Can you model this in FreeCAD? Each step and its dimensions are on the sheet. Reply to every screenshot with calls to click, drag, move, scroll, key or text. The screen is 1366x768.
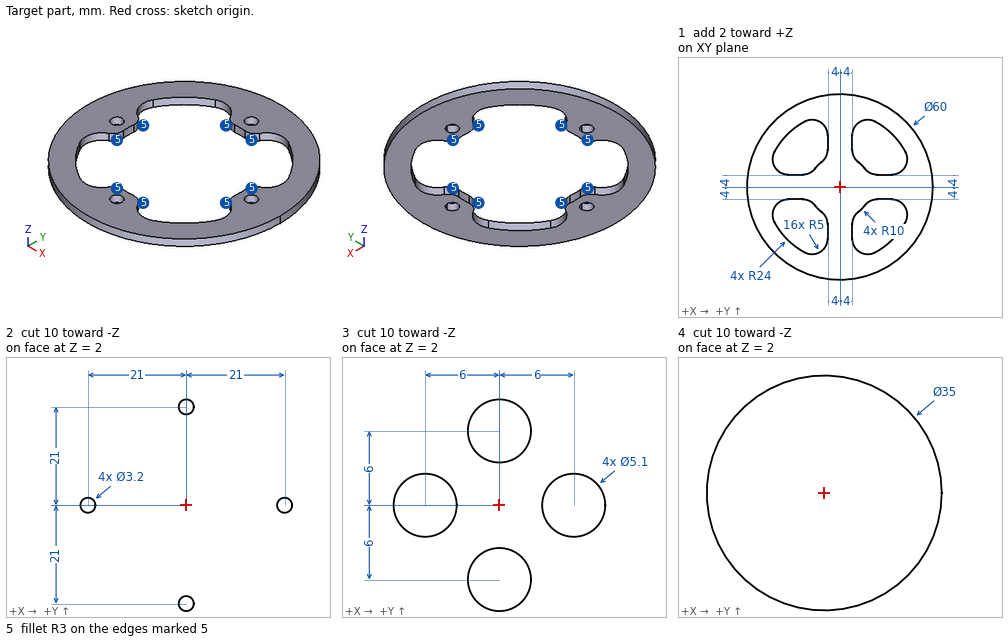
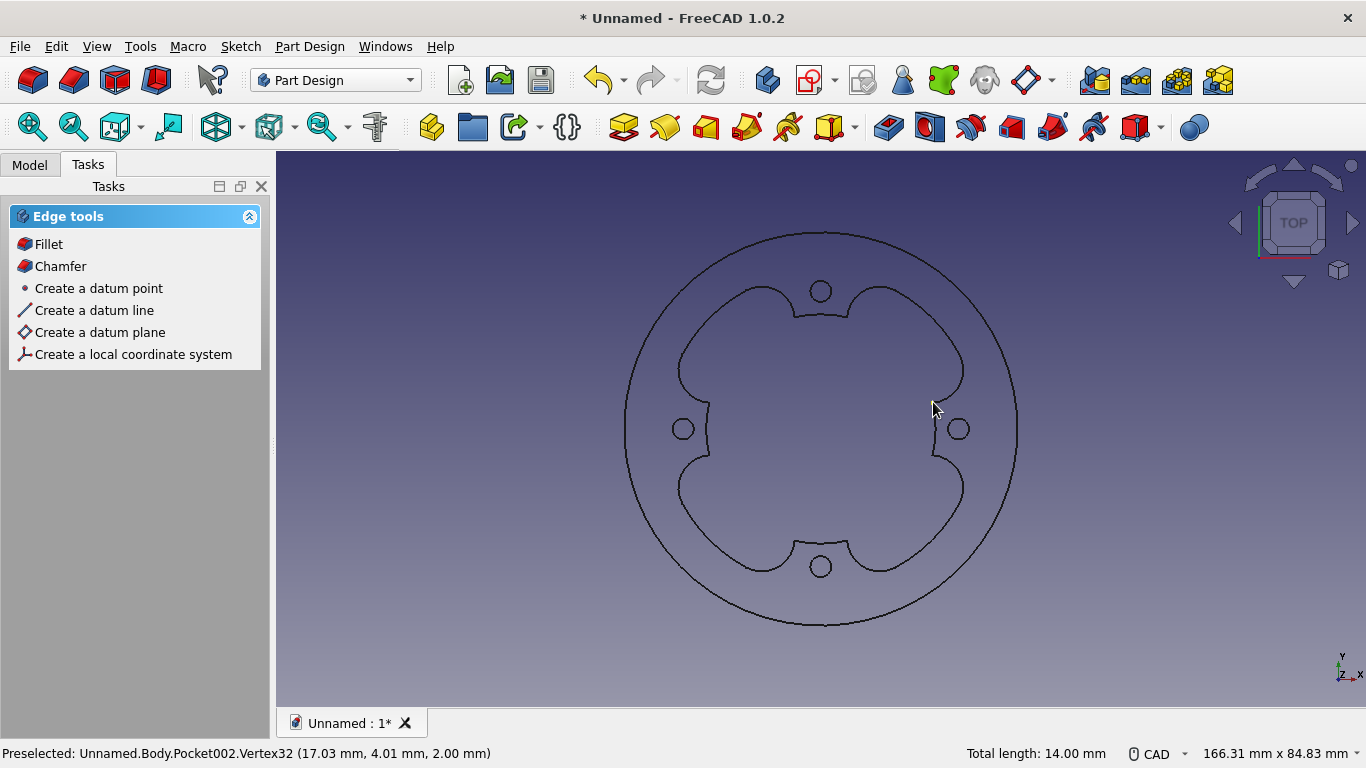
key(1)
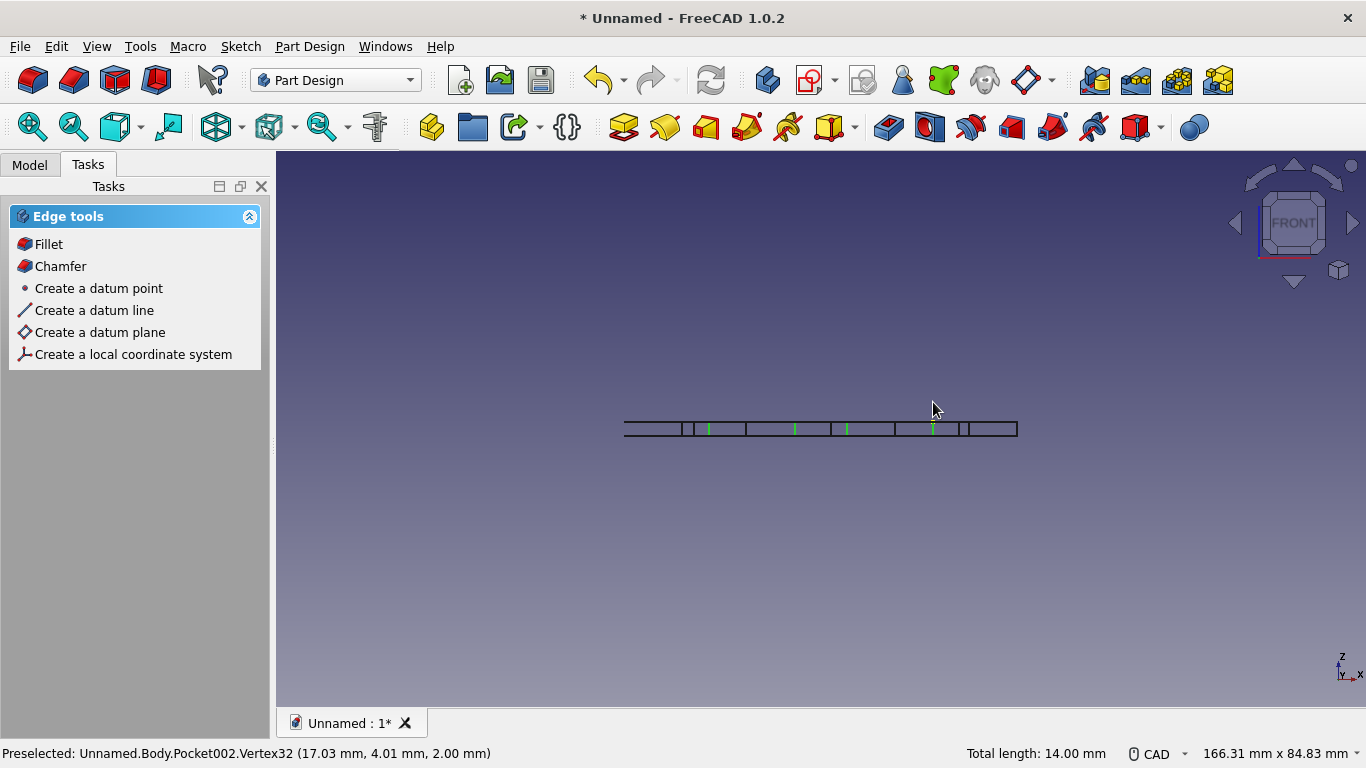
key(v)
key(f)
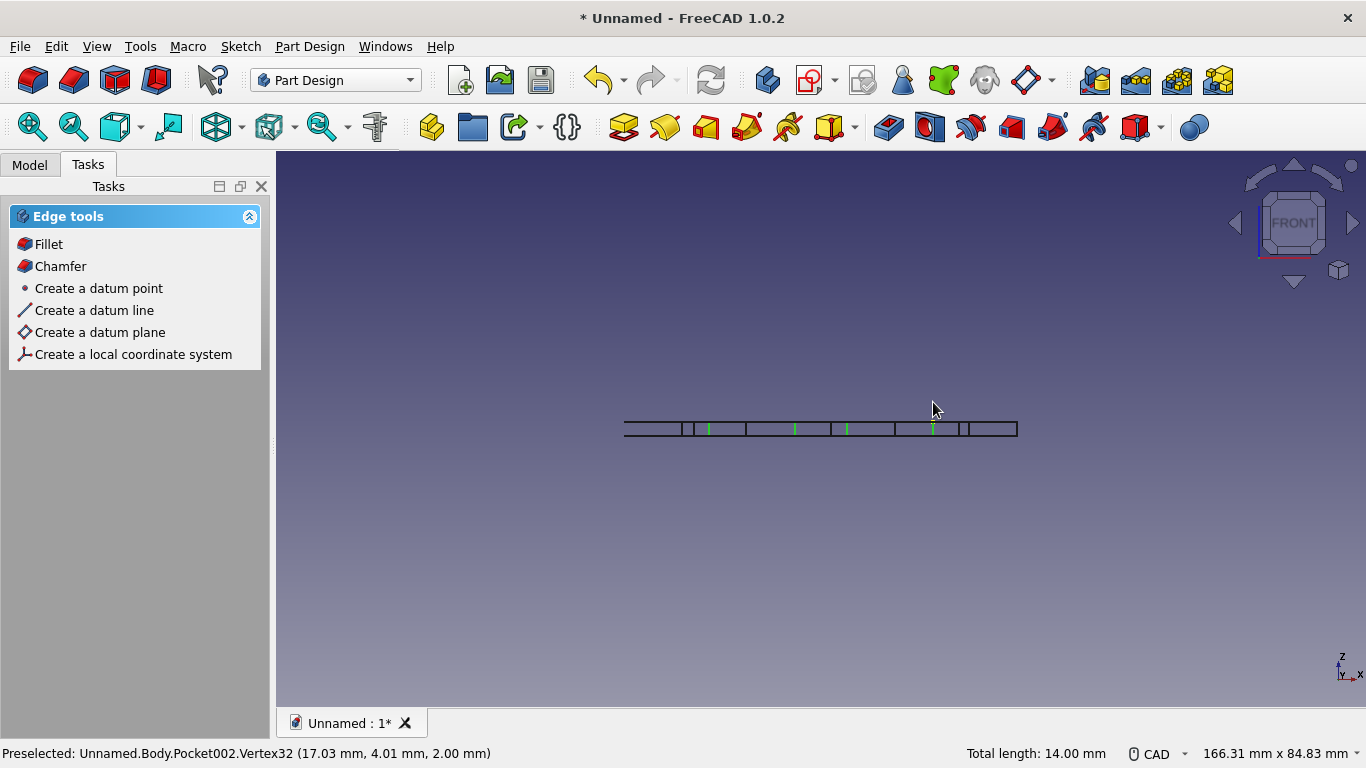
scroll(933, 428, up, 6)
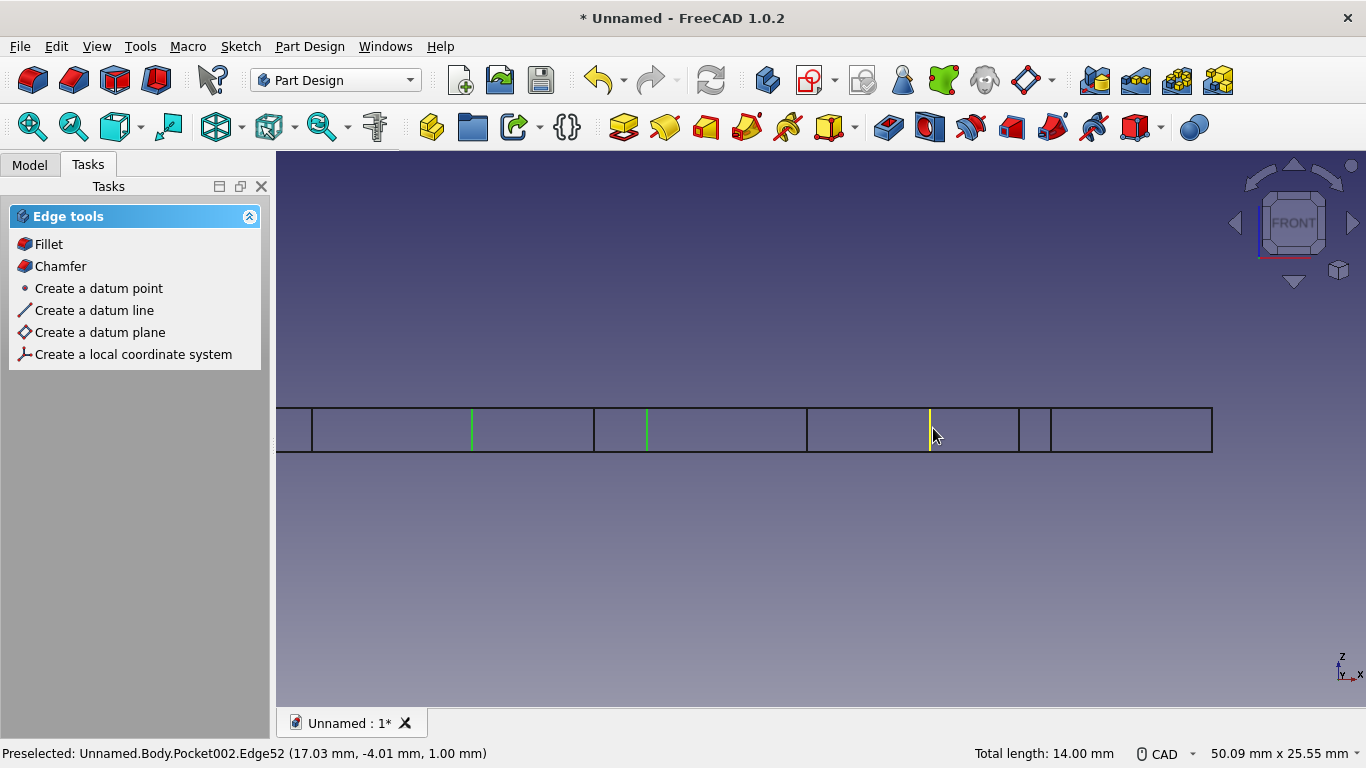
key(v)
key(f)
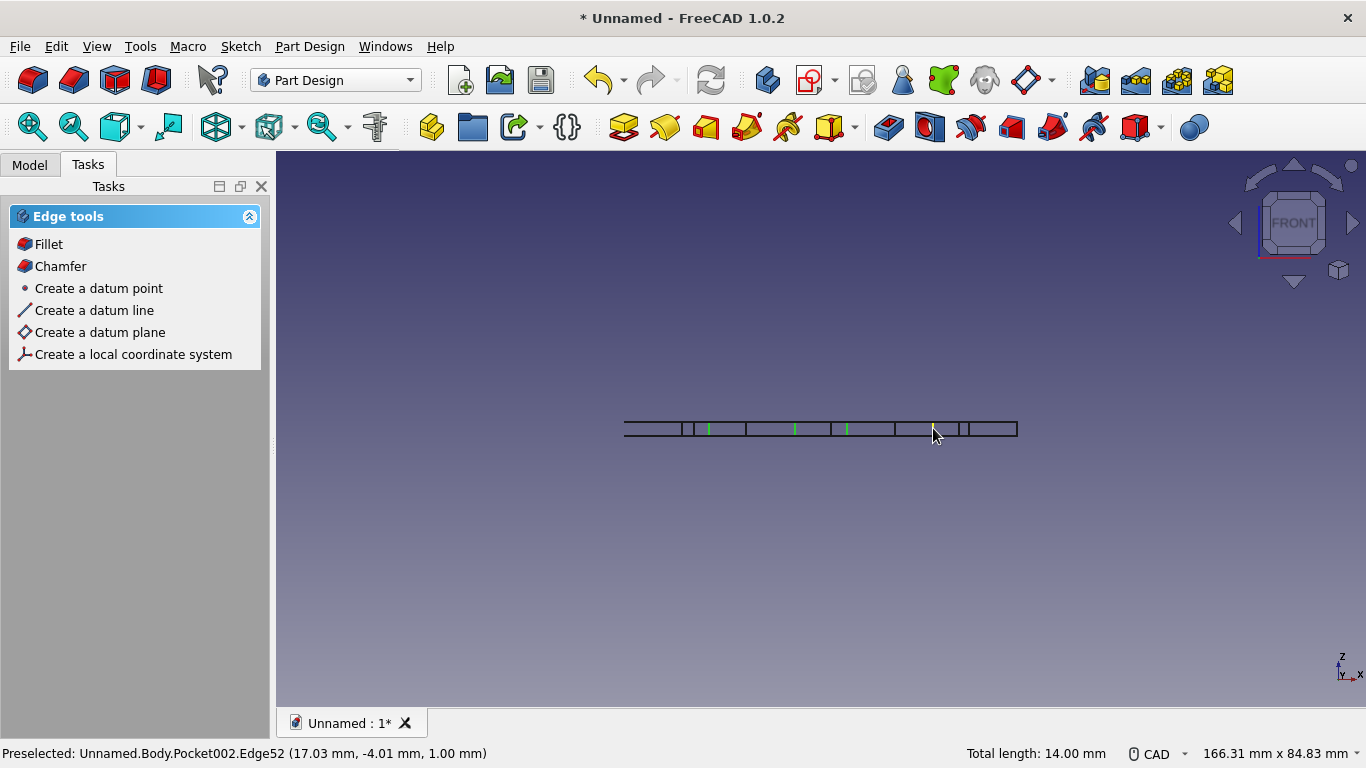
key(3)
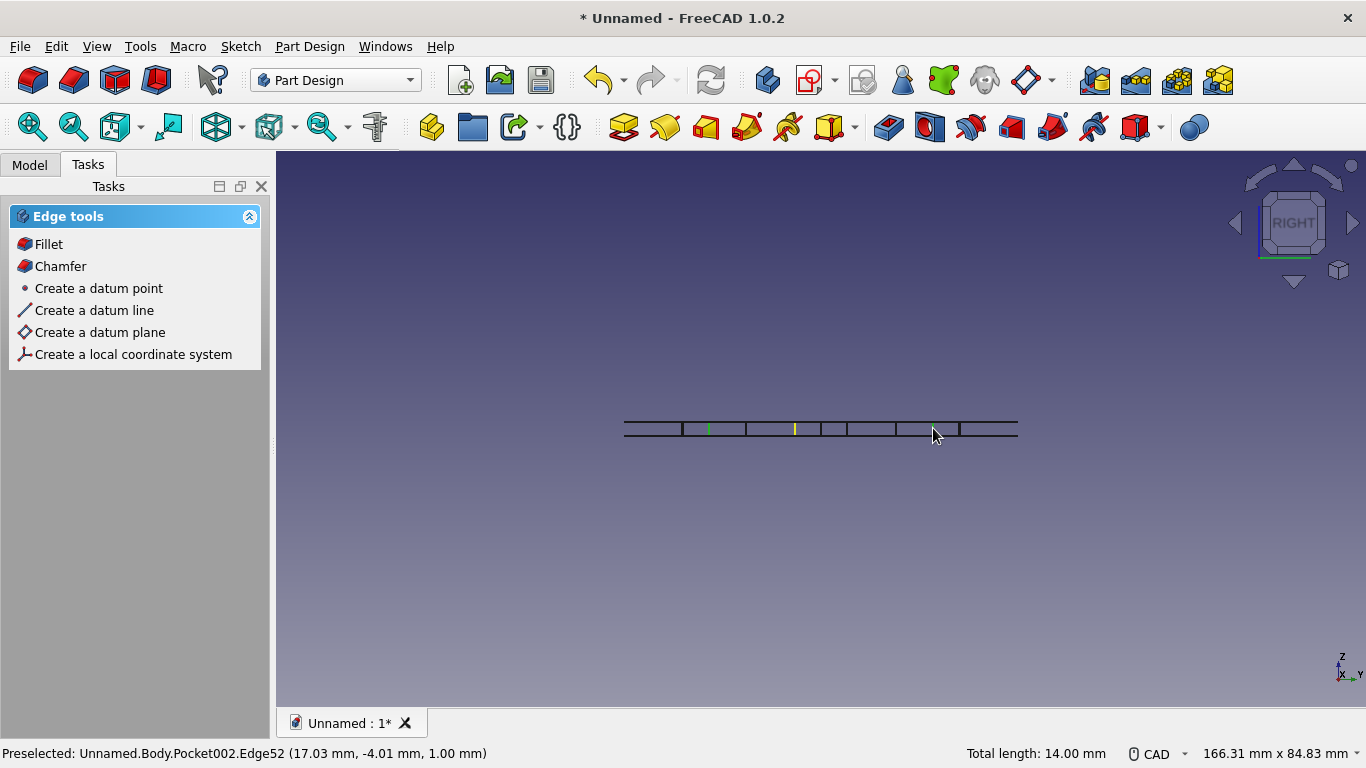
key(v)
key(f)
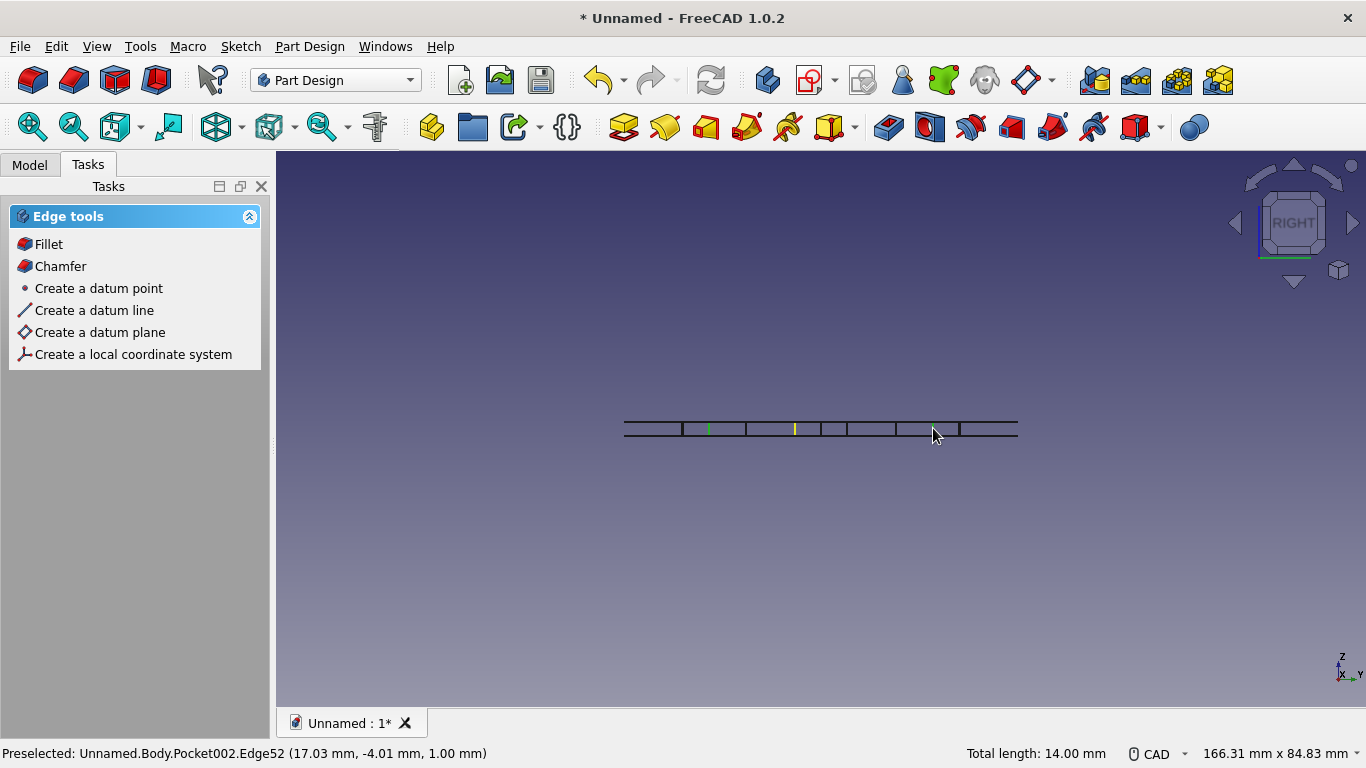
click(847, 428, ctrl)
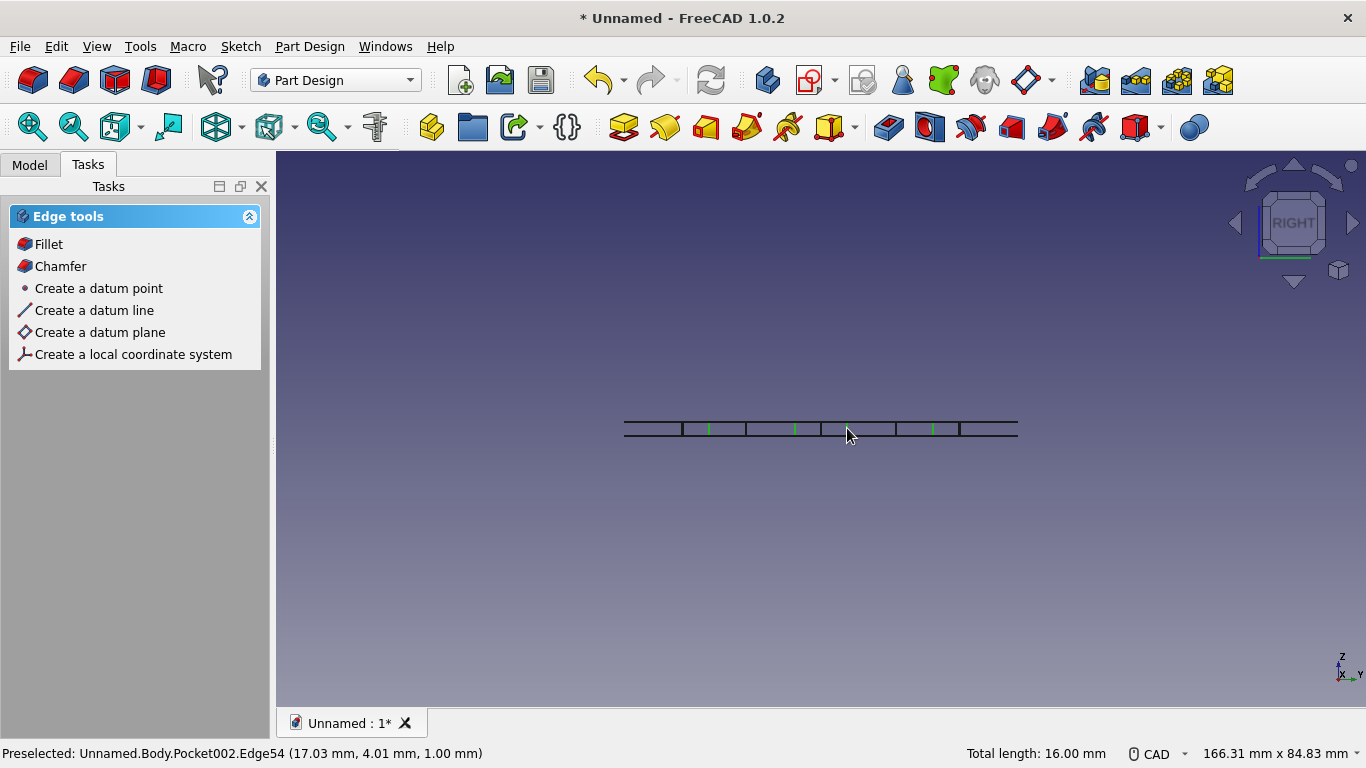
key(v)
key(1)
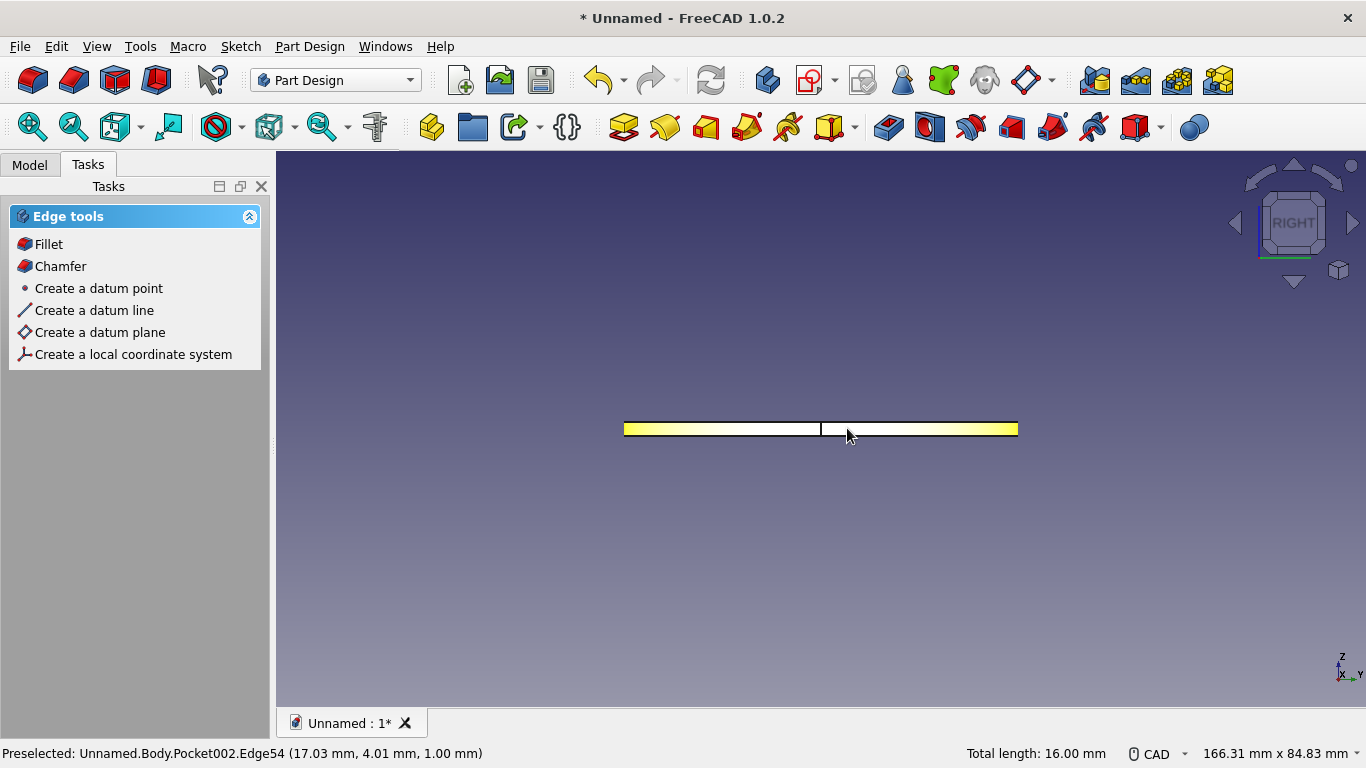
click(33, 80)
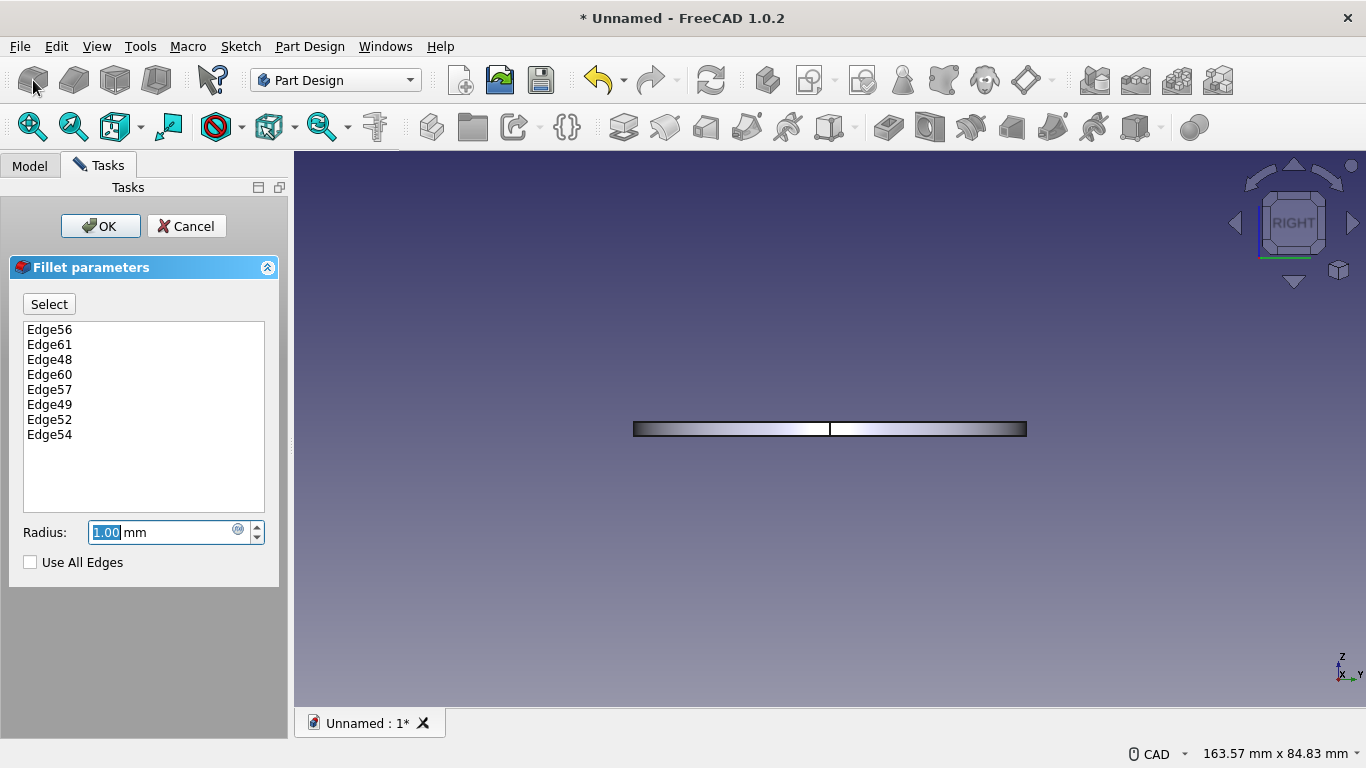
text(3)
key(Tab)